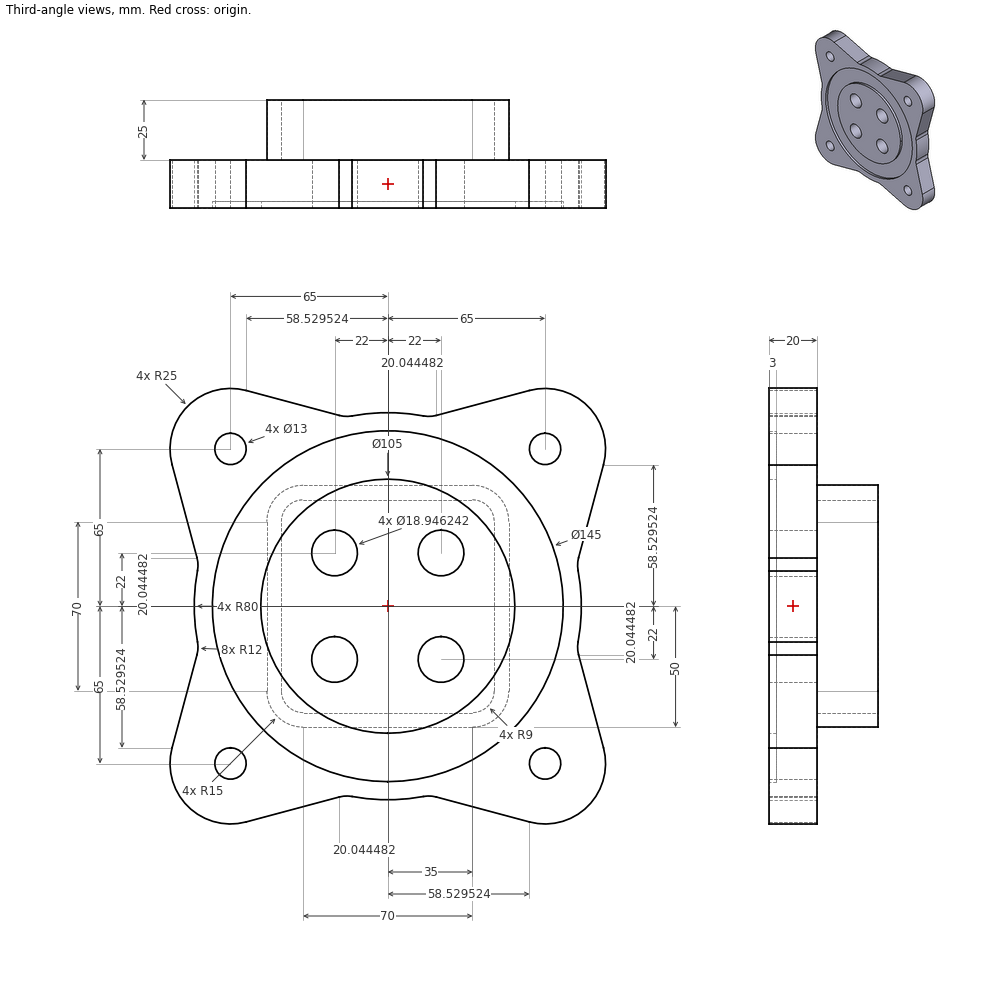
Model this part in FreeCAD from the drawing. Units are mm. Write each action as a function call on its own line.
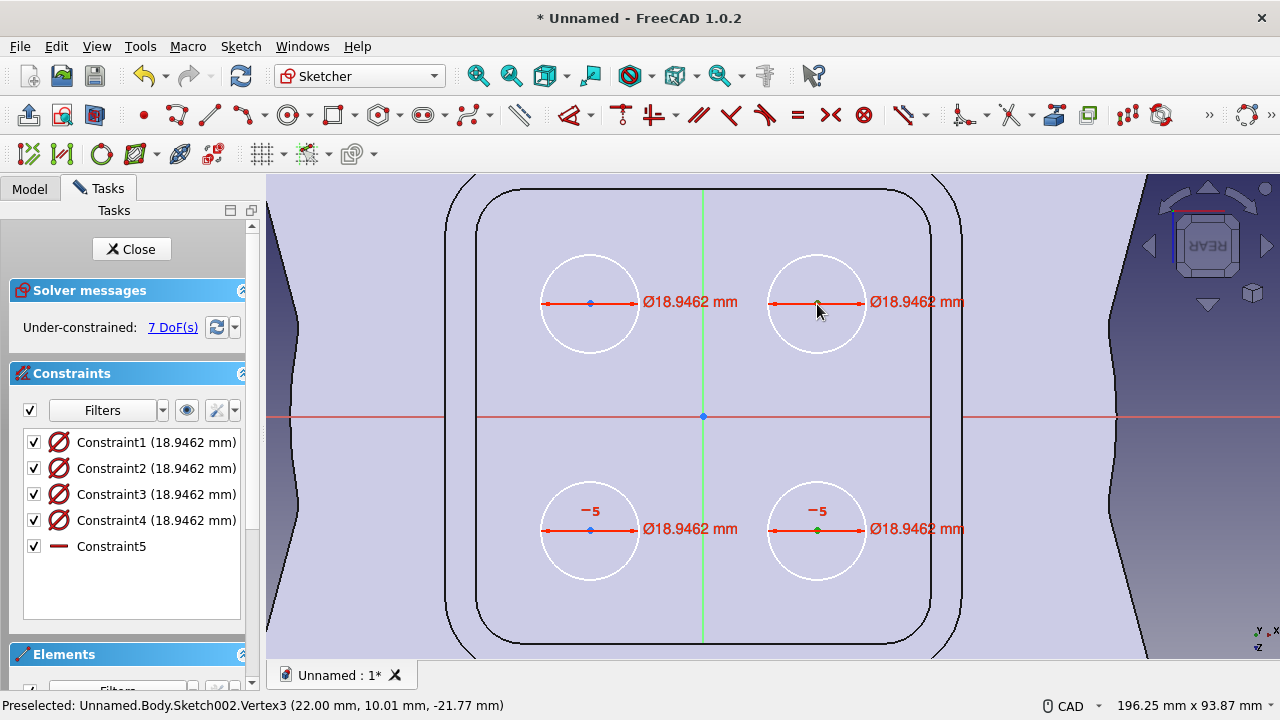
key(v)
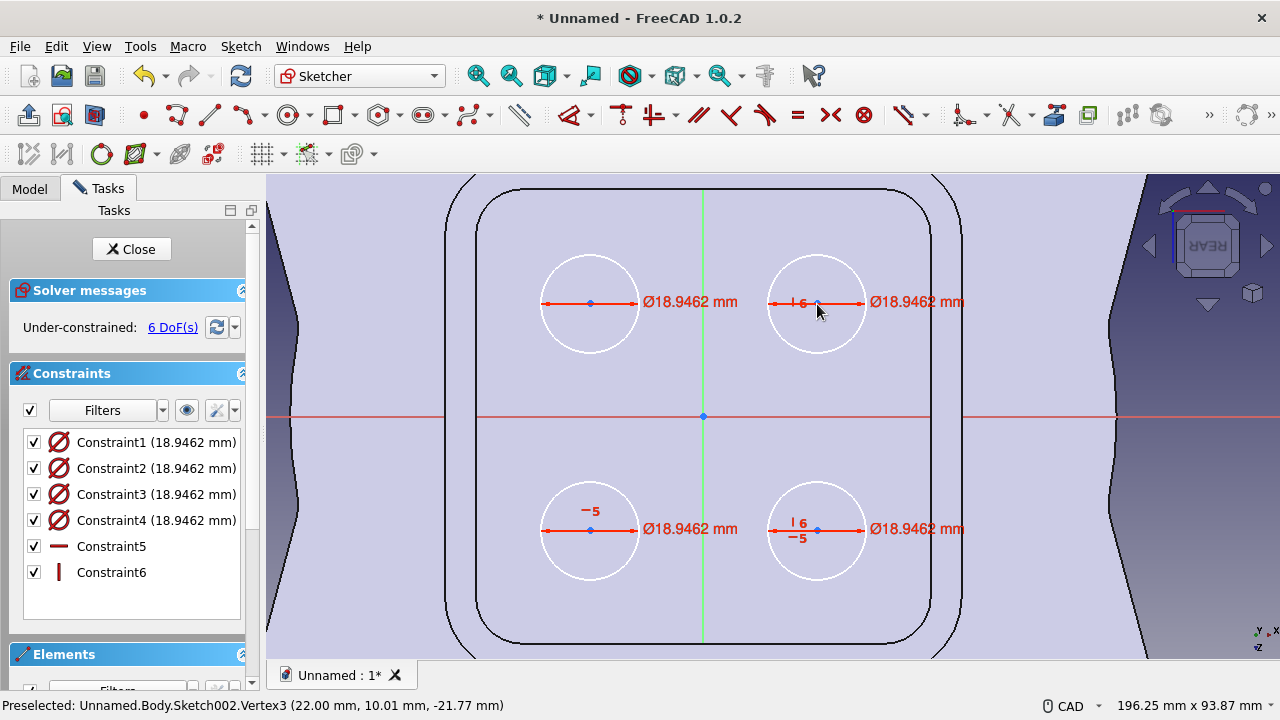
click(590, 531)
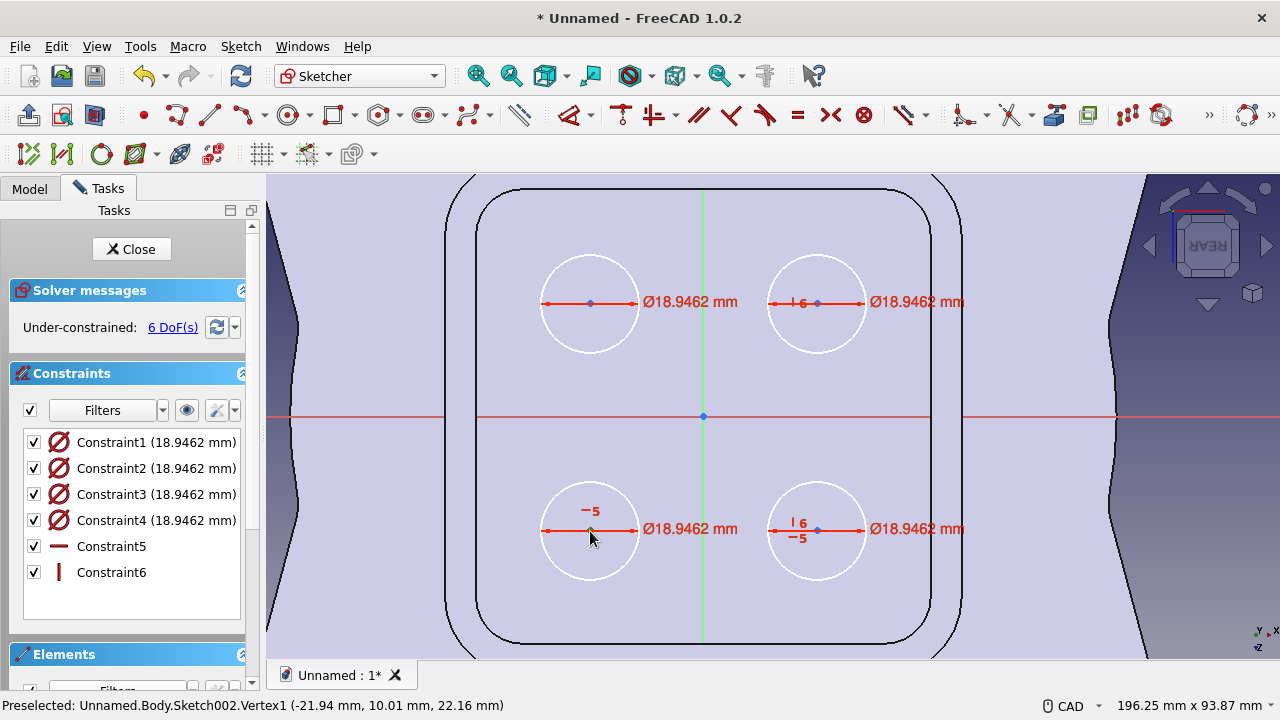
click(590, 304)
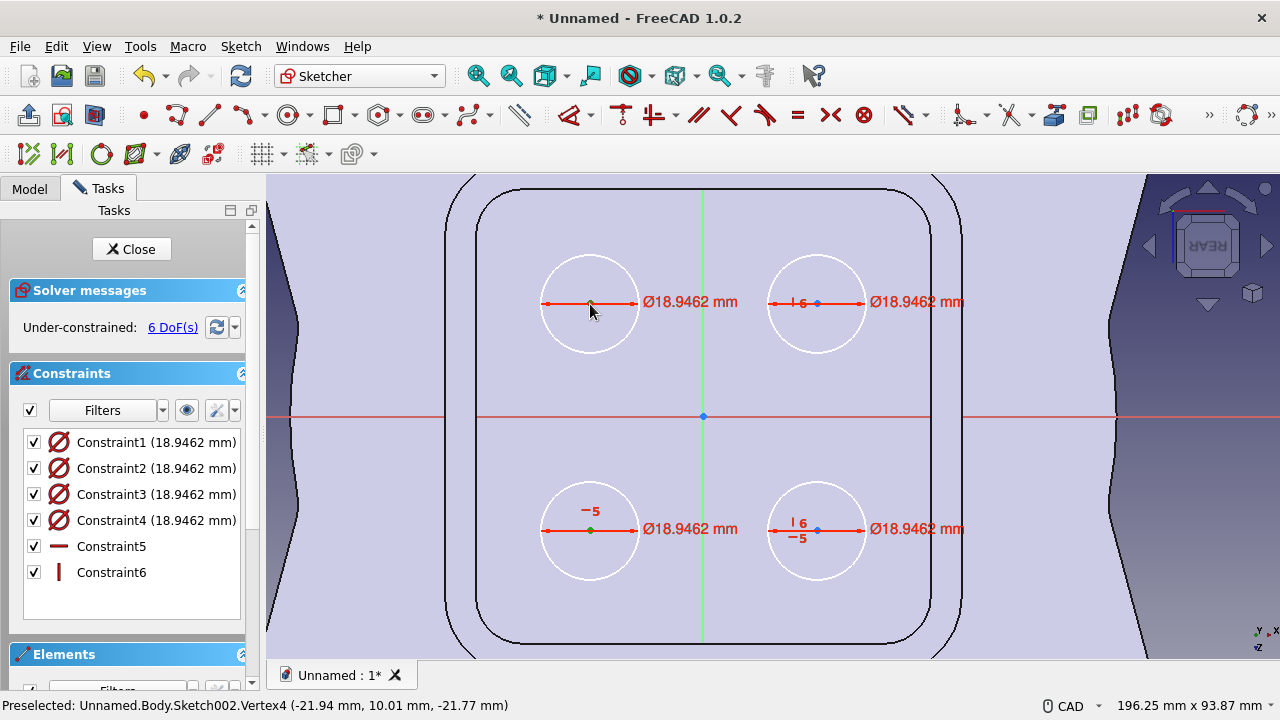
key(v)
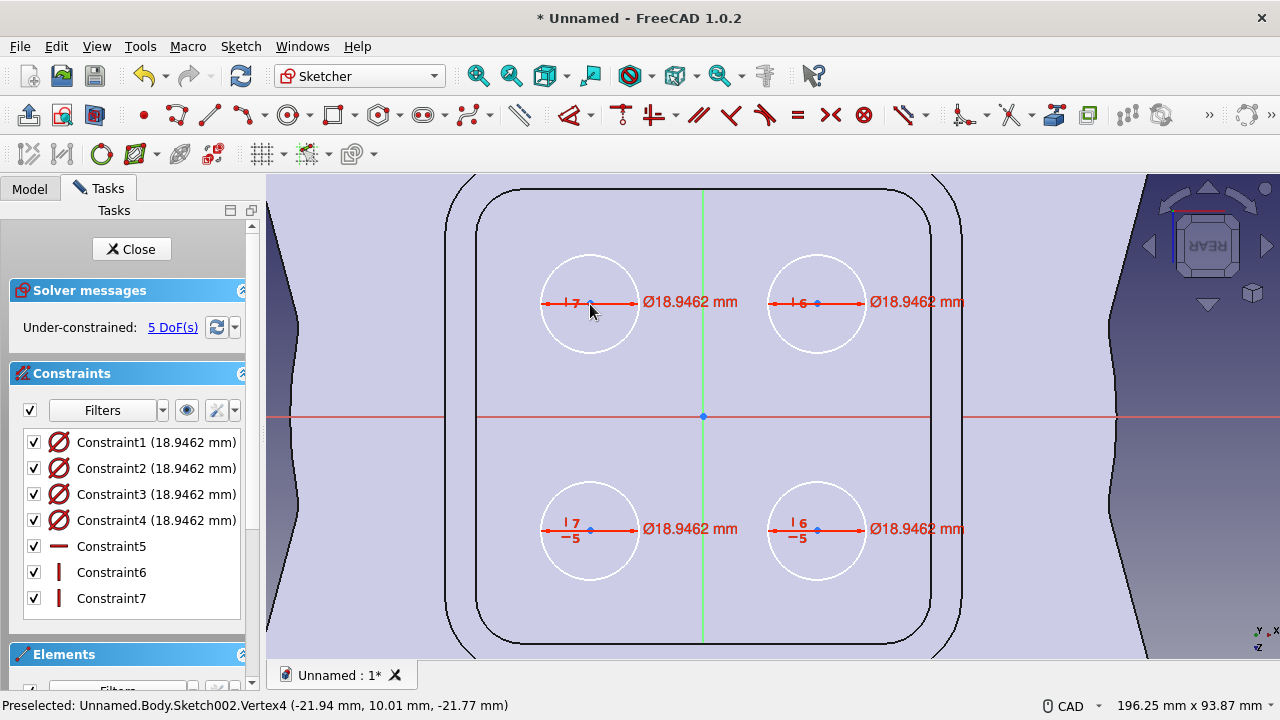
click(817, 304)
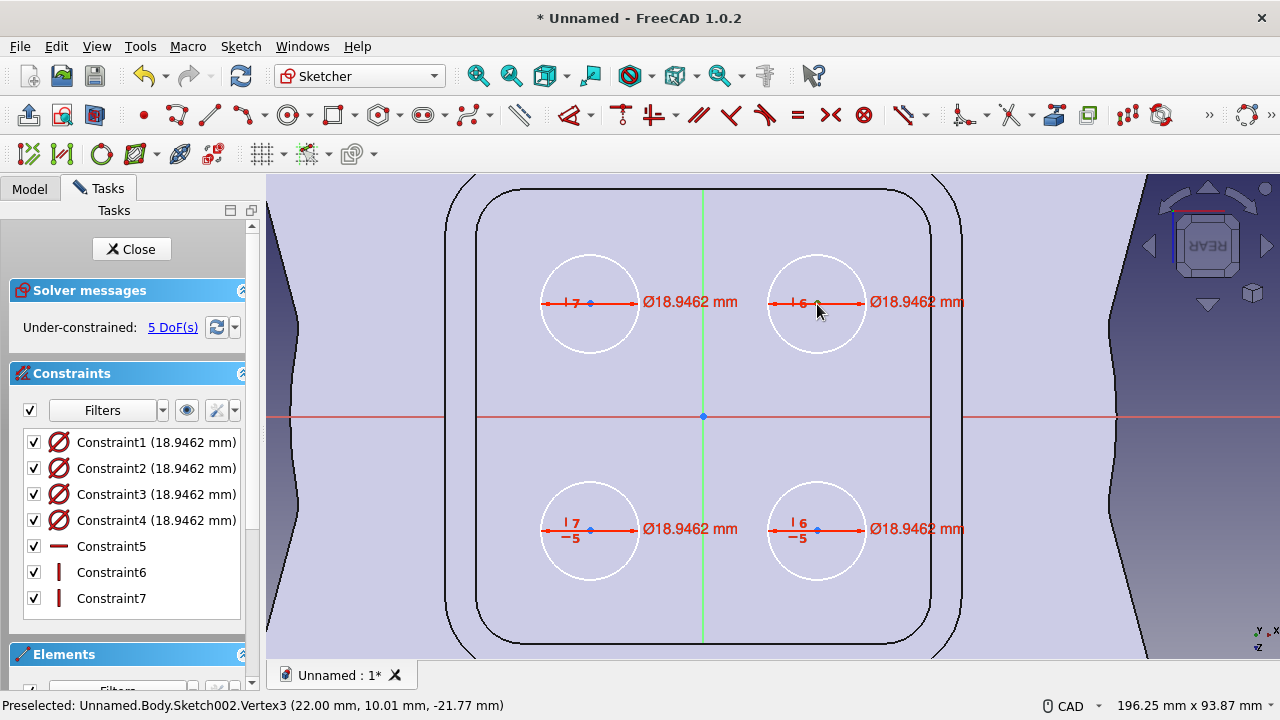
click(590, 304)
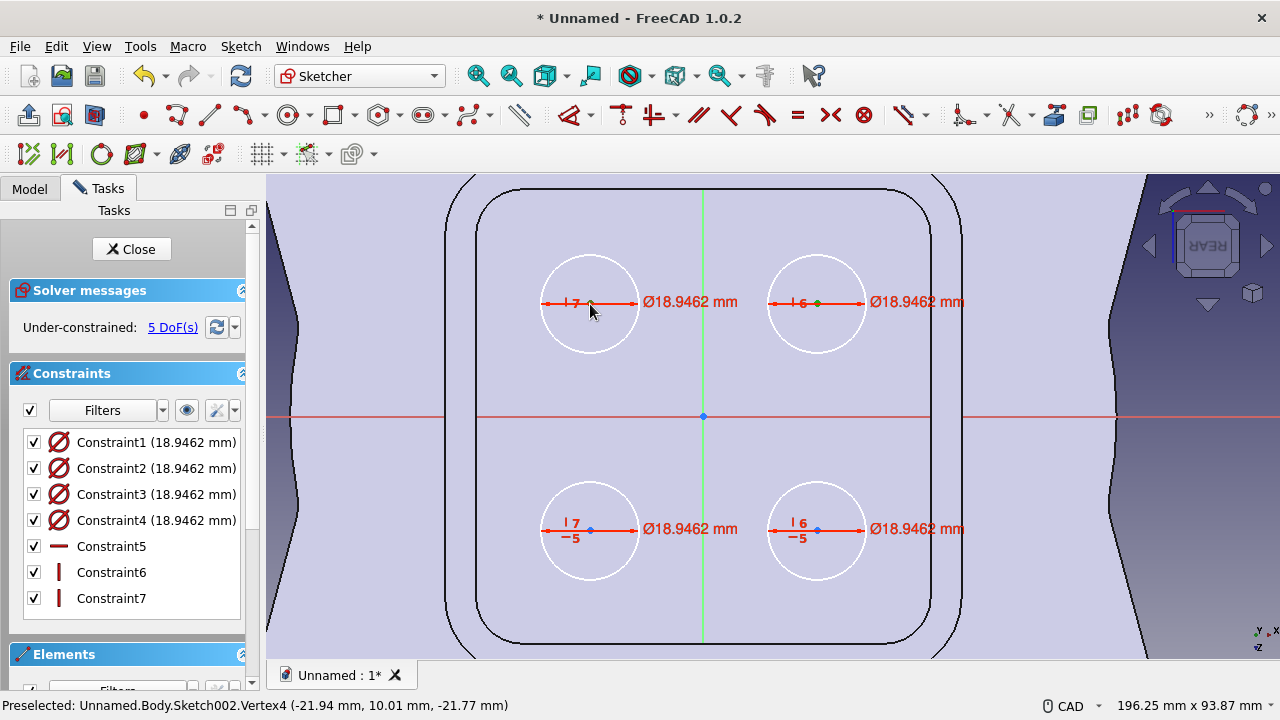
key(h)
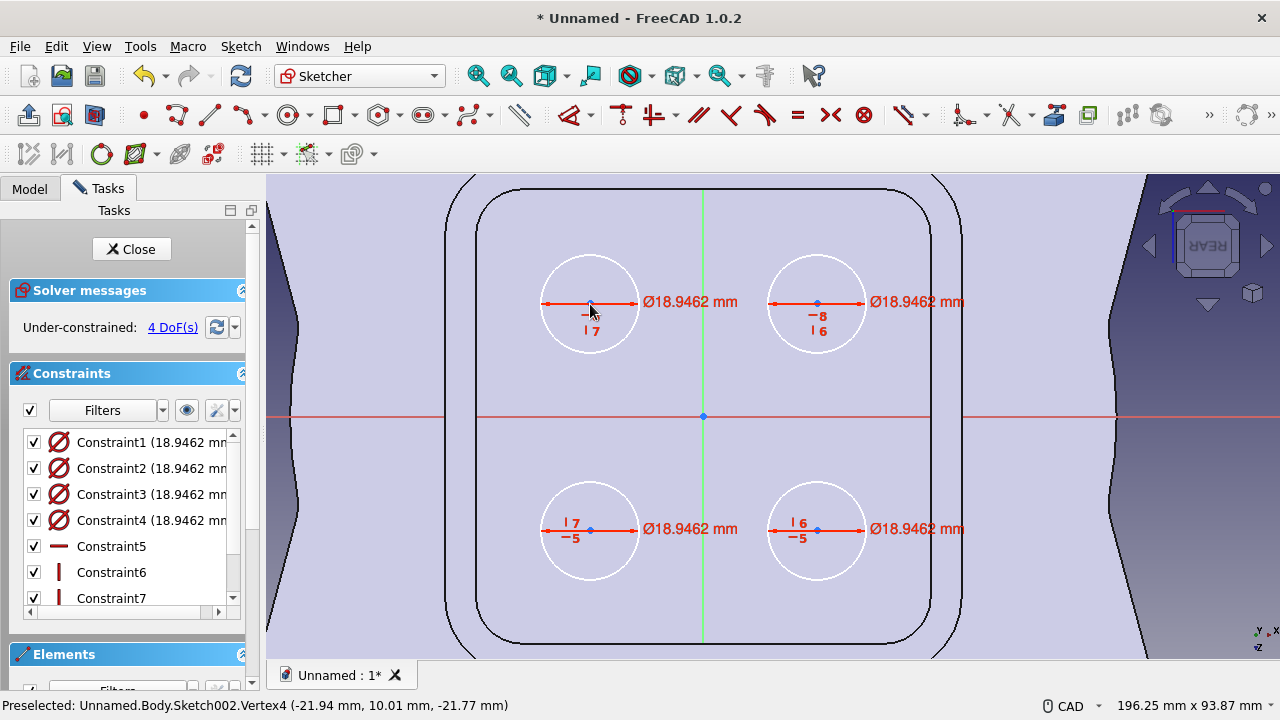
key(d)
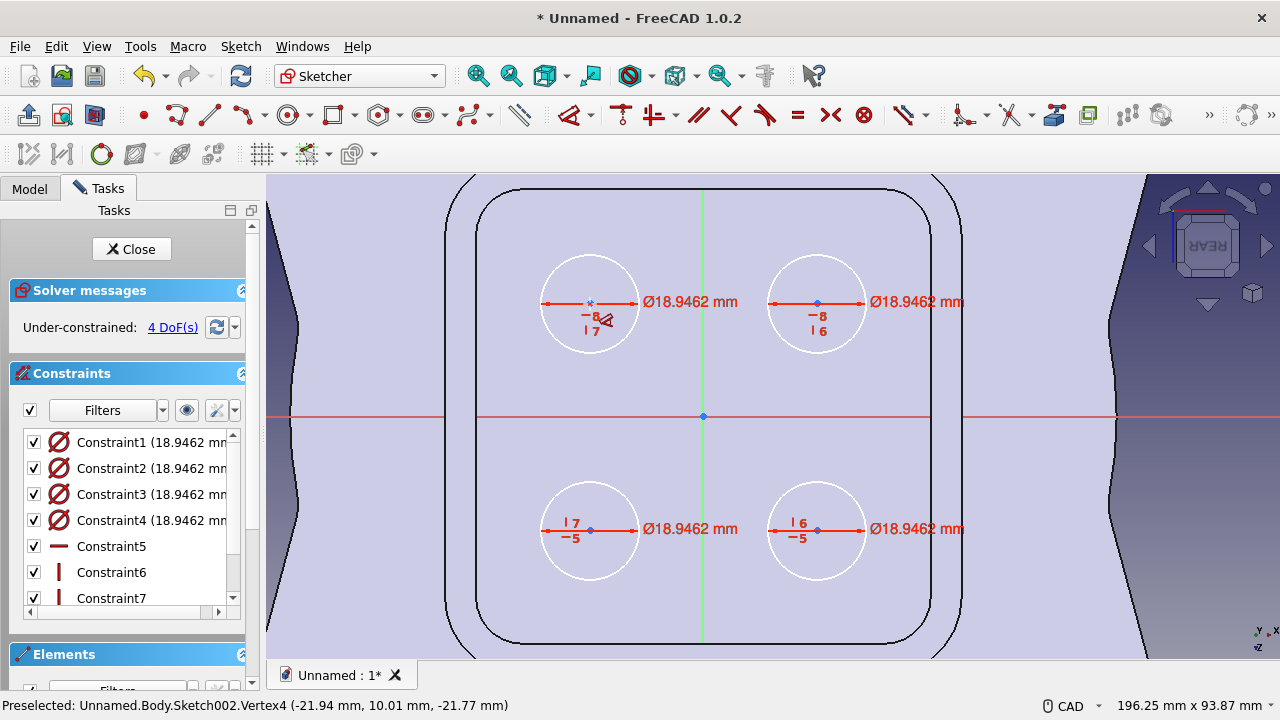
click(590, 531)
click(647, 565)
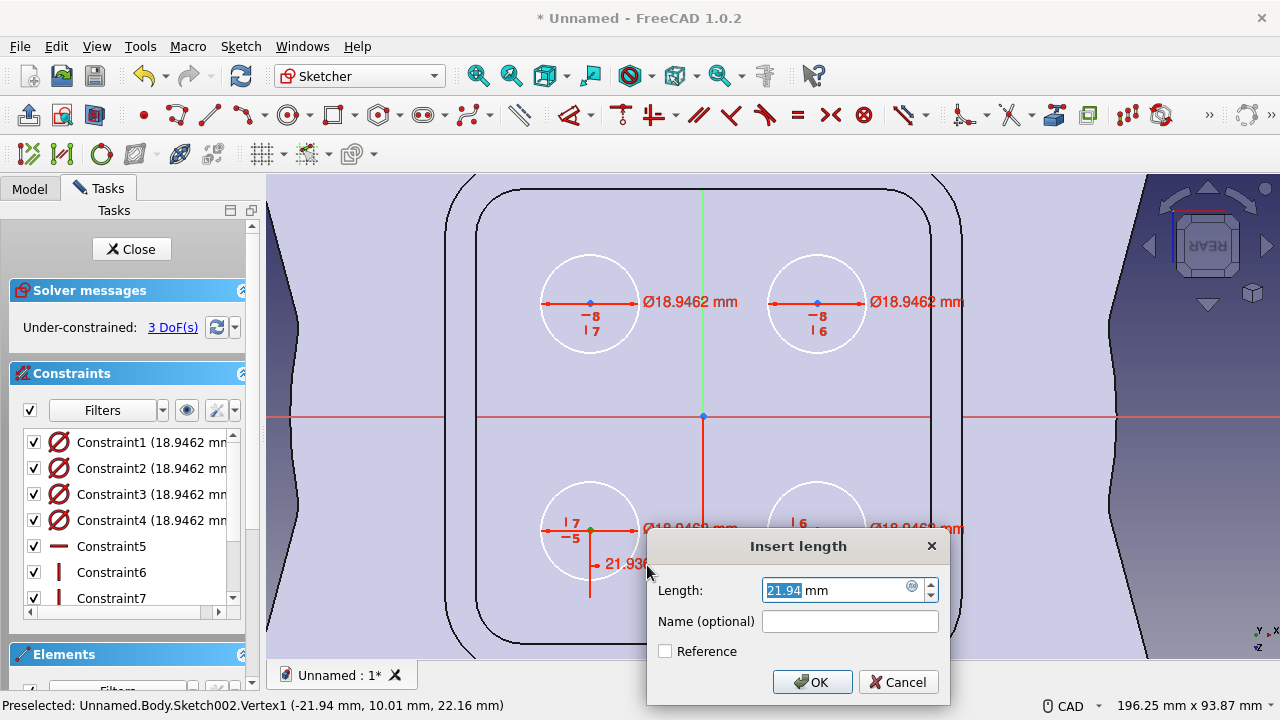
text(22)
key(Return)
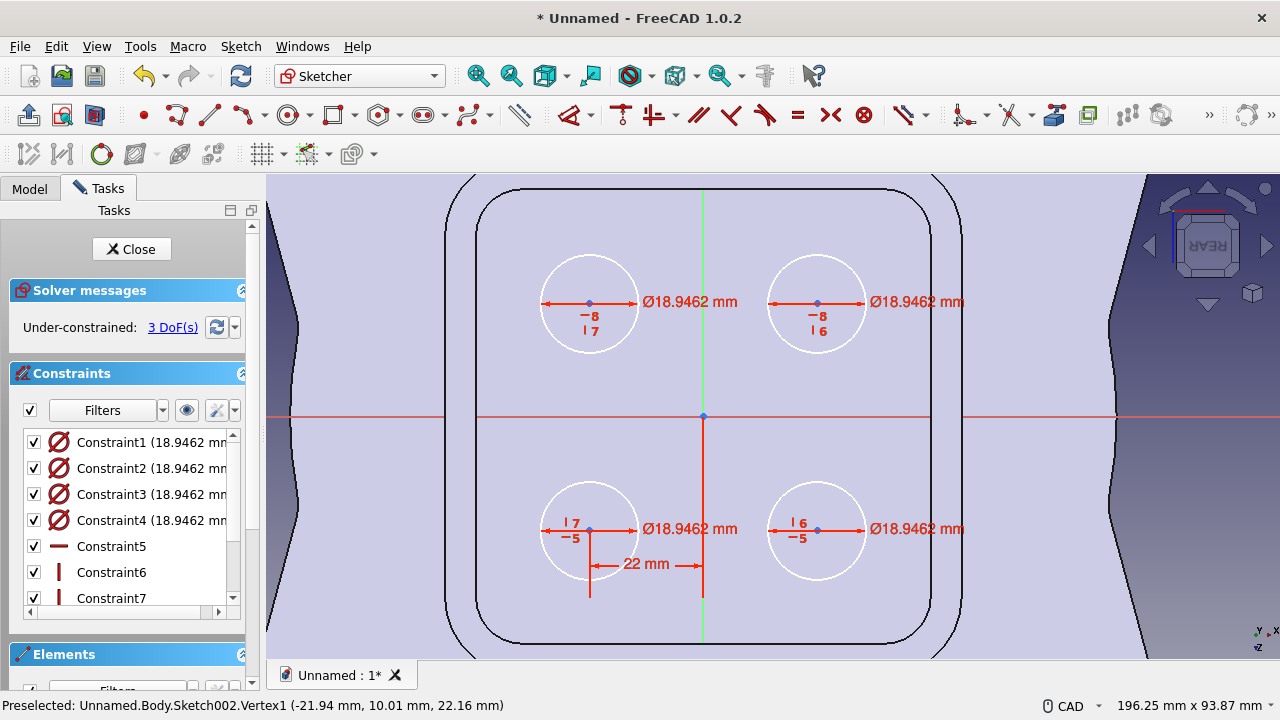
click(590, 531)
click(556, 474)